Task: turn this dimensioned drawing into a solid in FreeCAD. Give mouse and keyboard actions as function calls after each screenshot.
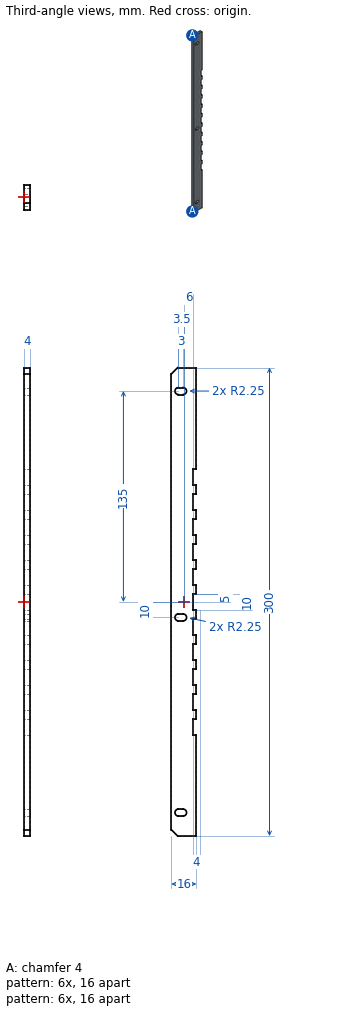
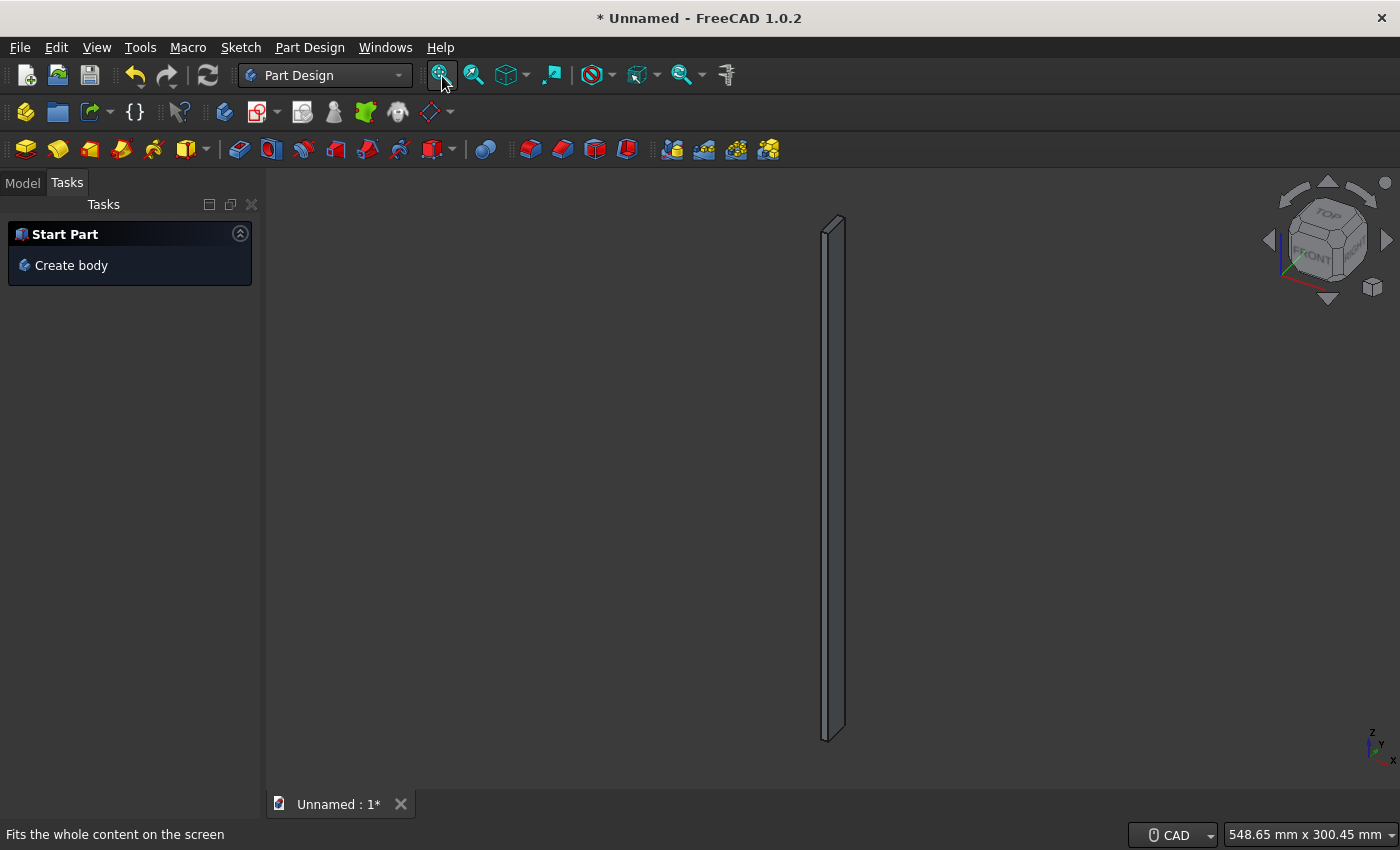
key(0)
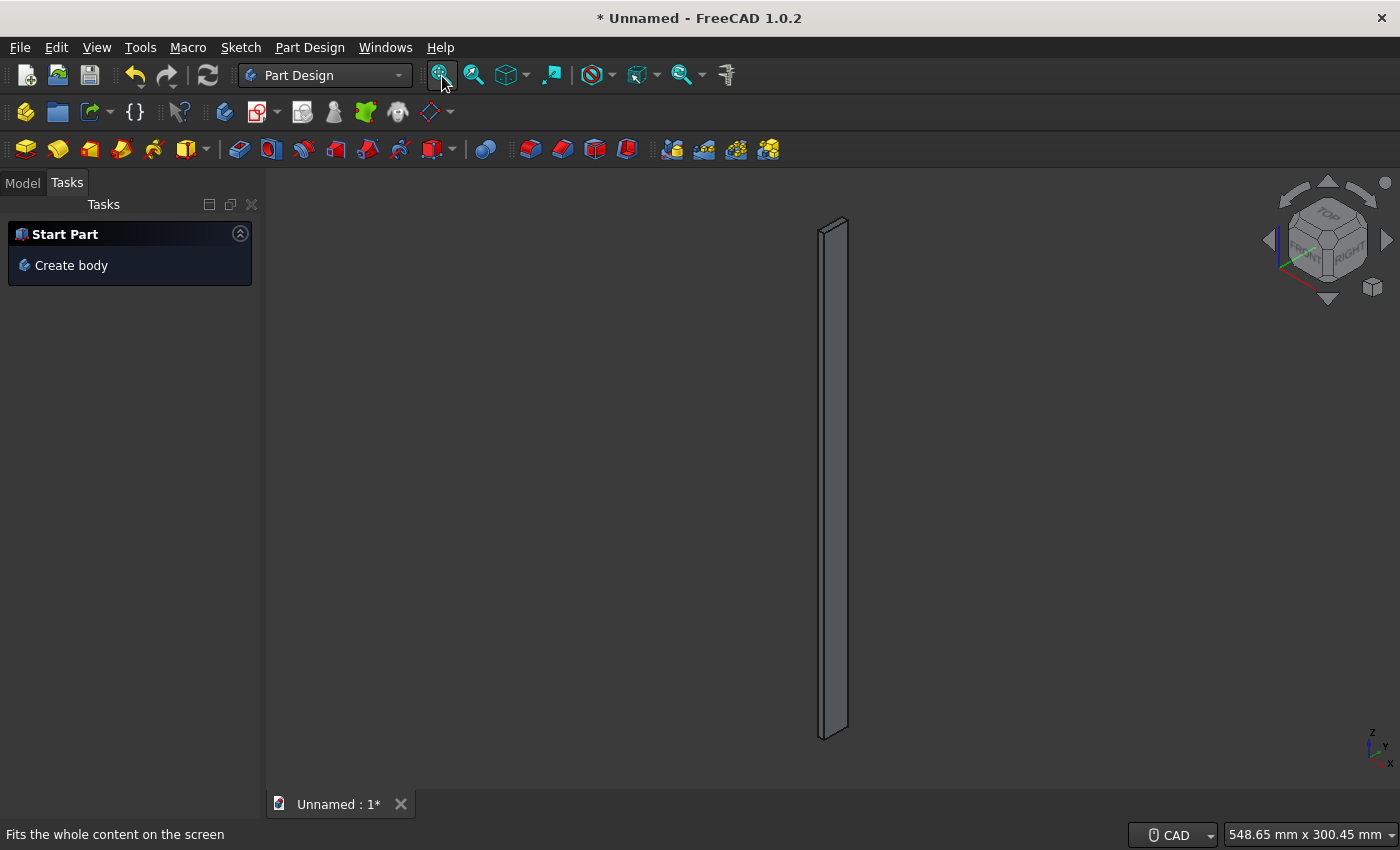
scroll(821, 737, up, 8)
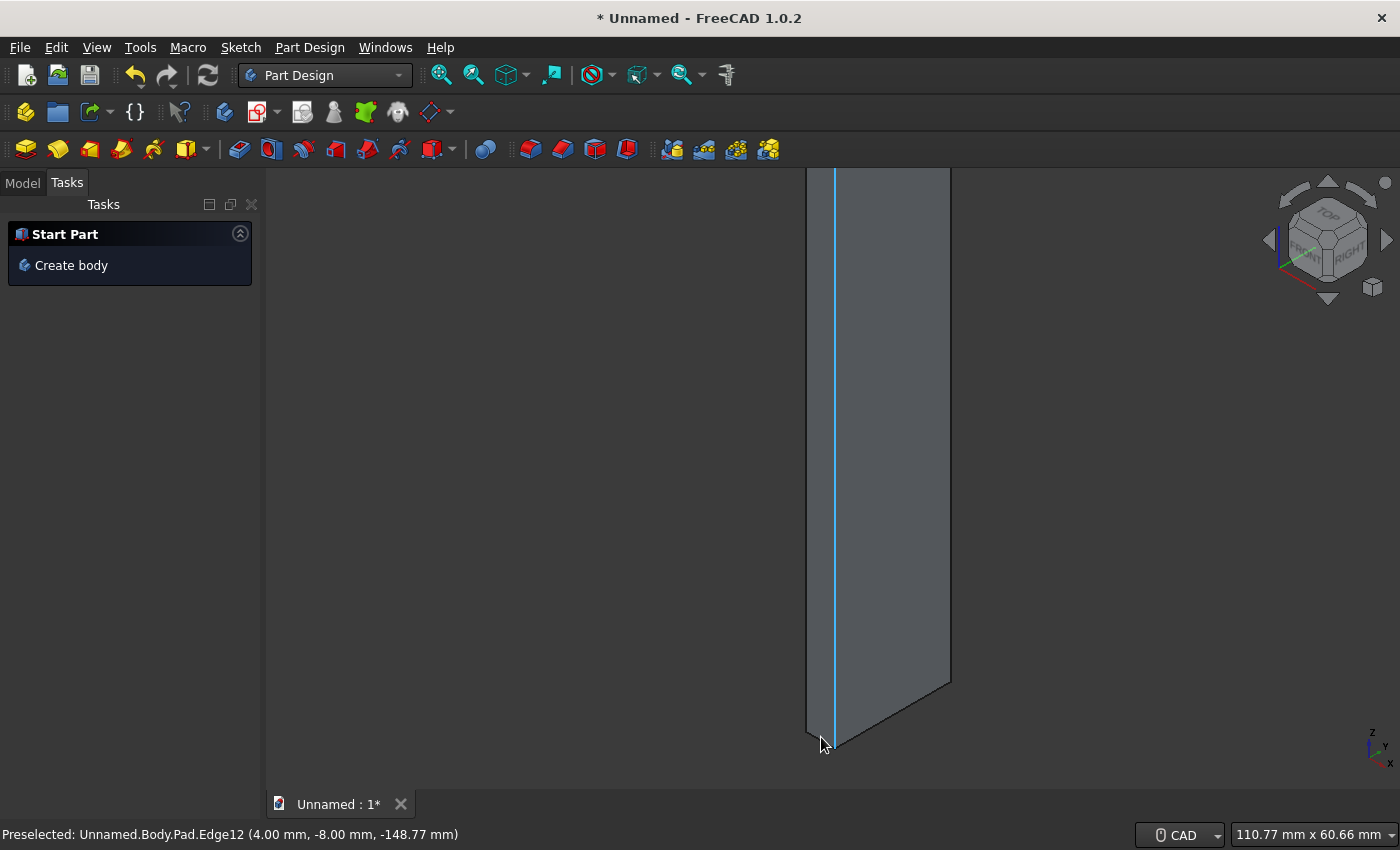
click(442, 76)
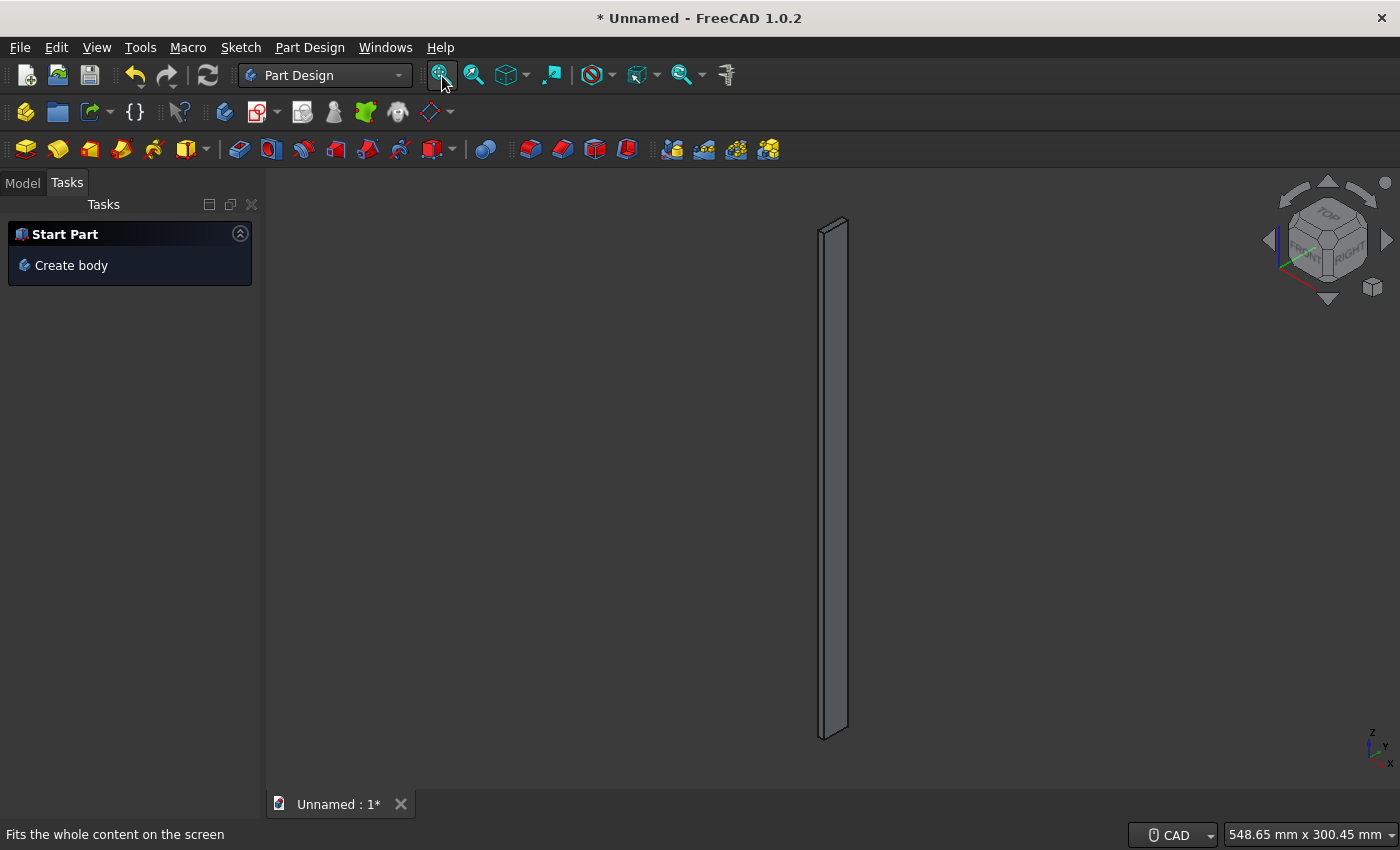
key(2)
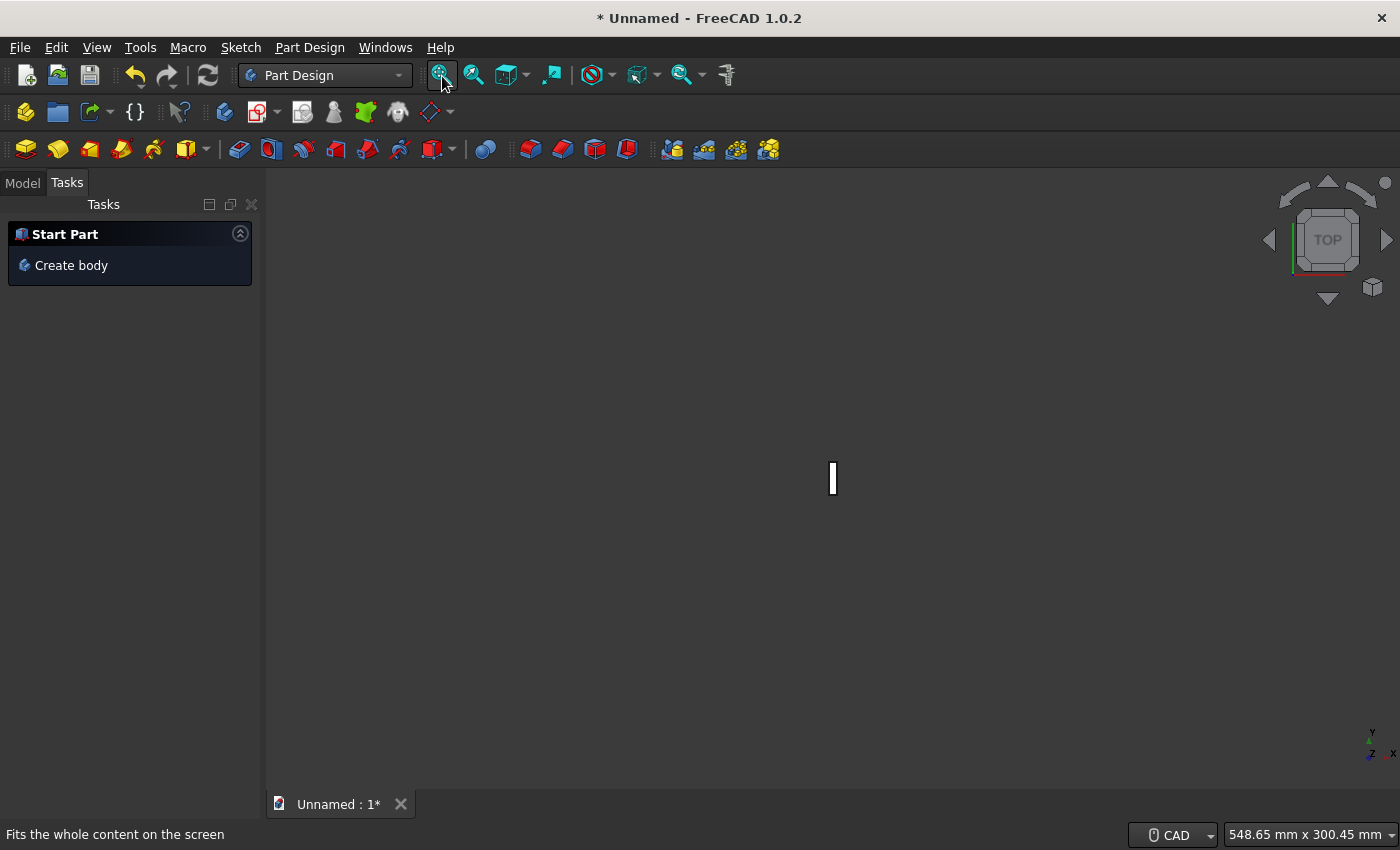
key(v)
key(f)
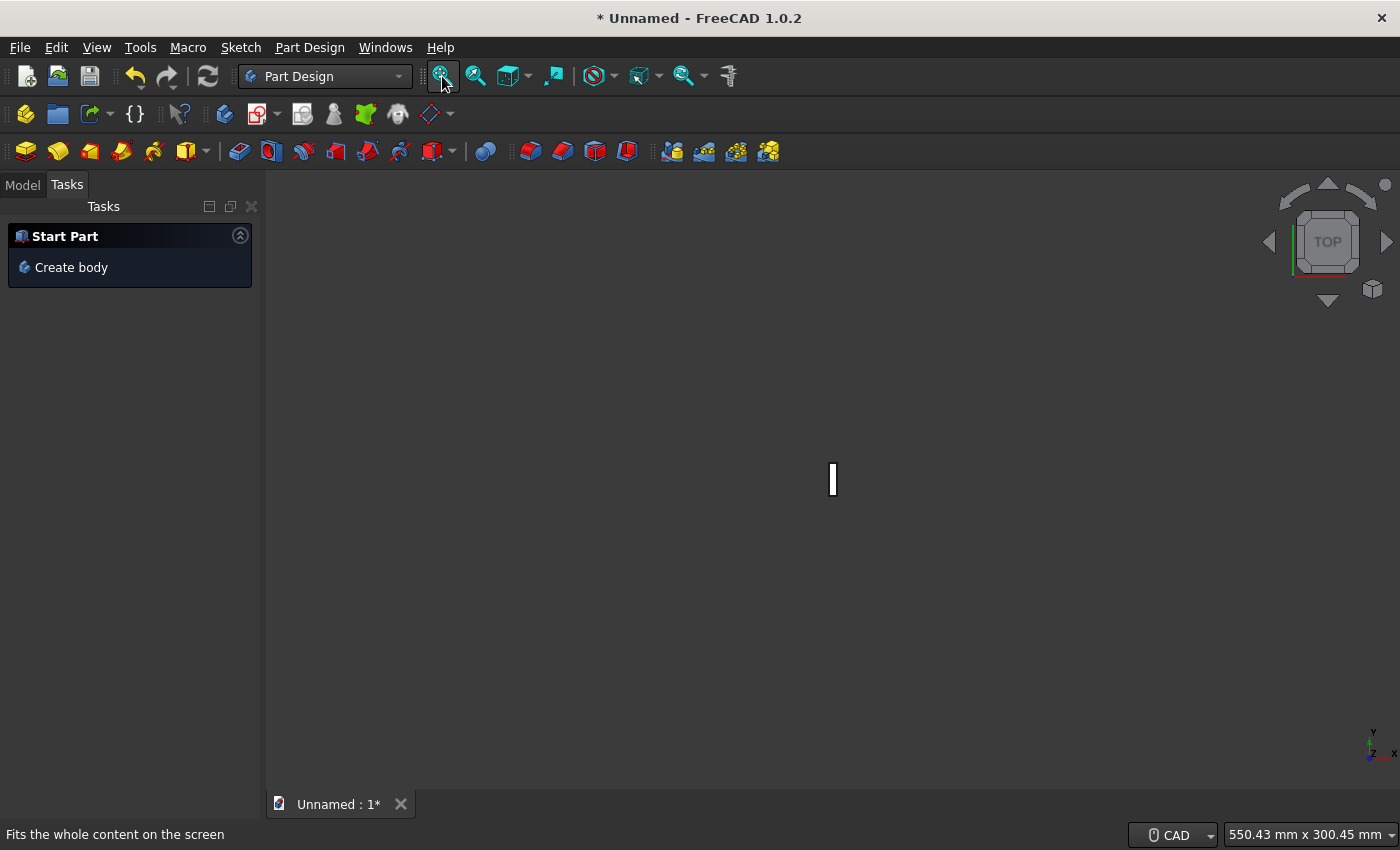
scroll(833, 495, up, 8)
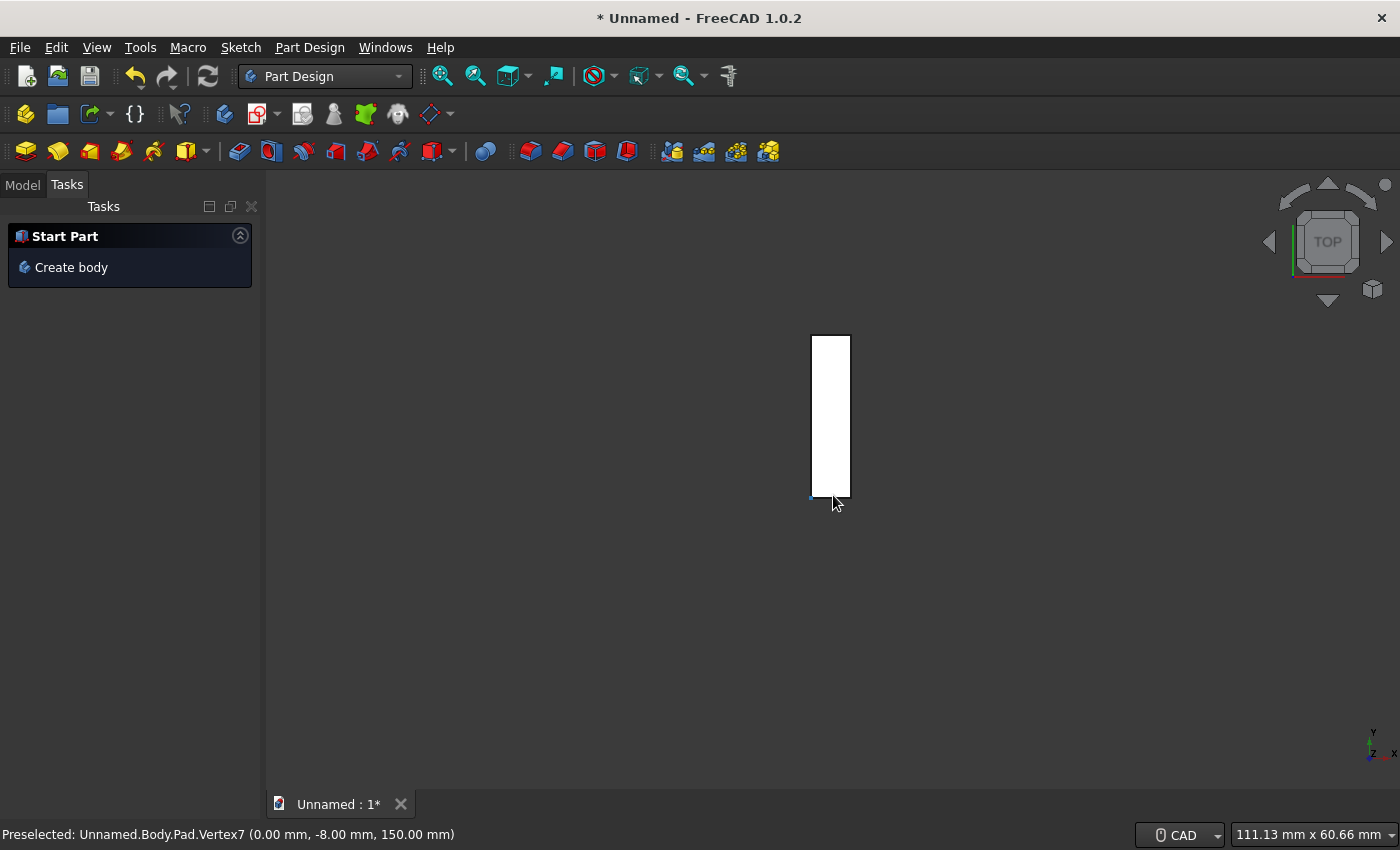
click(831, 497)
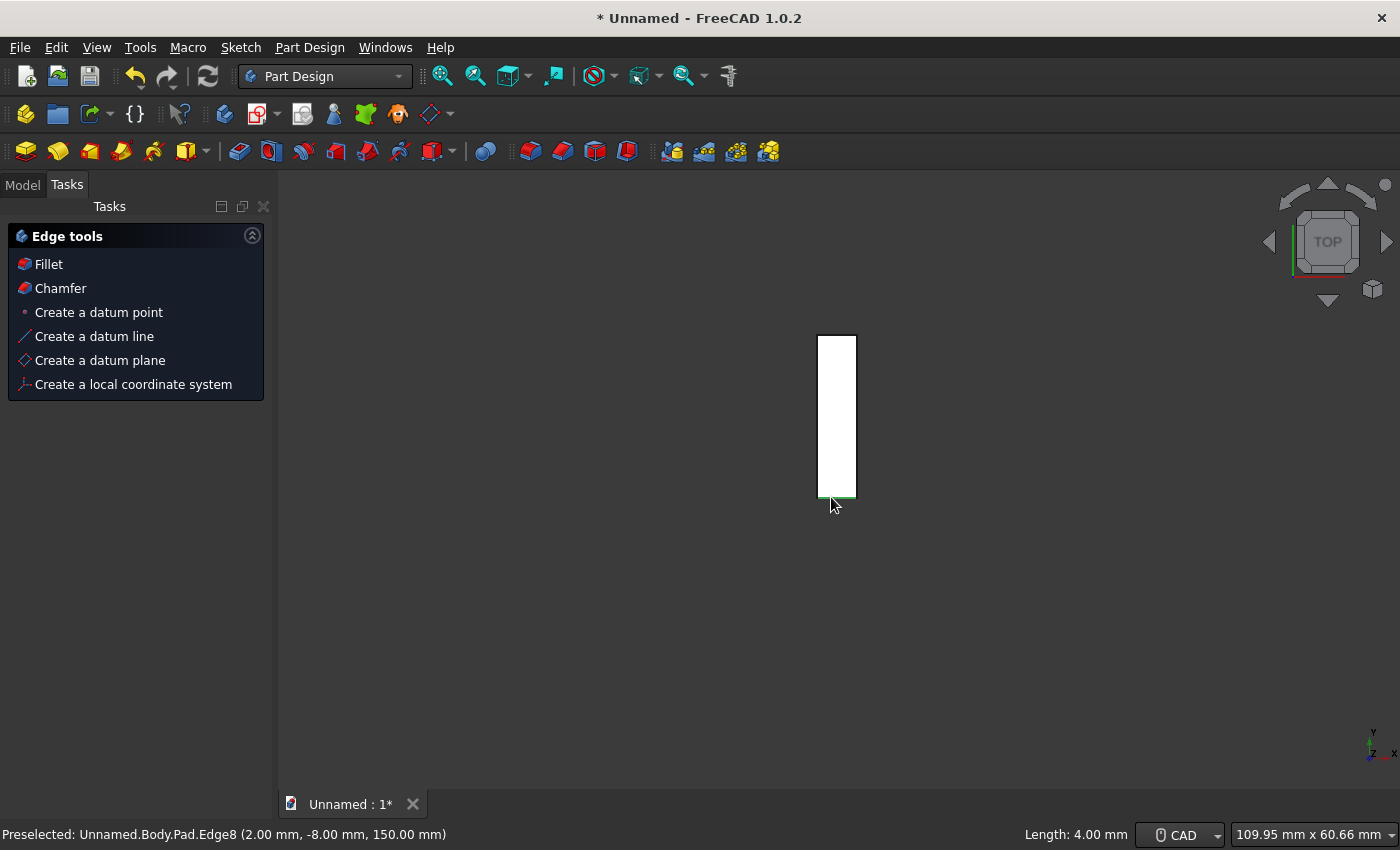
key(v)
key(f)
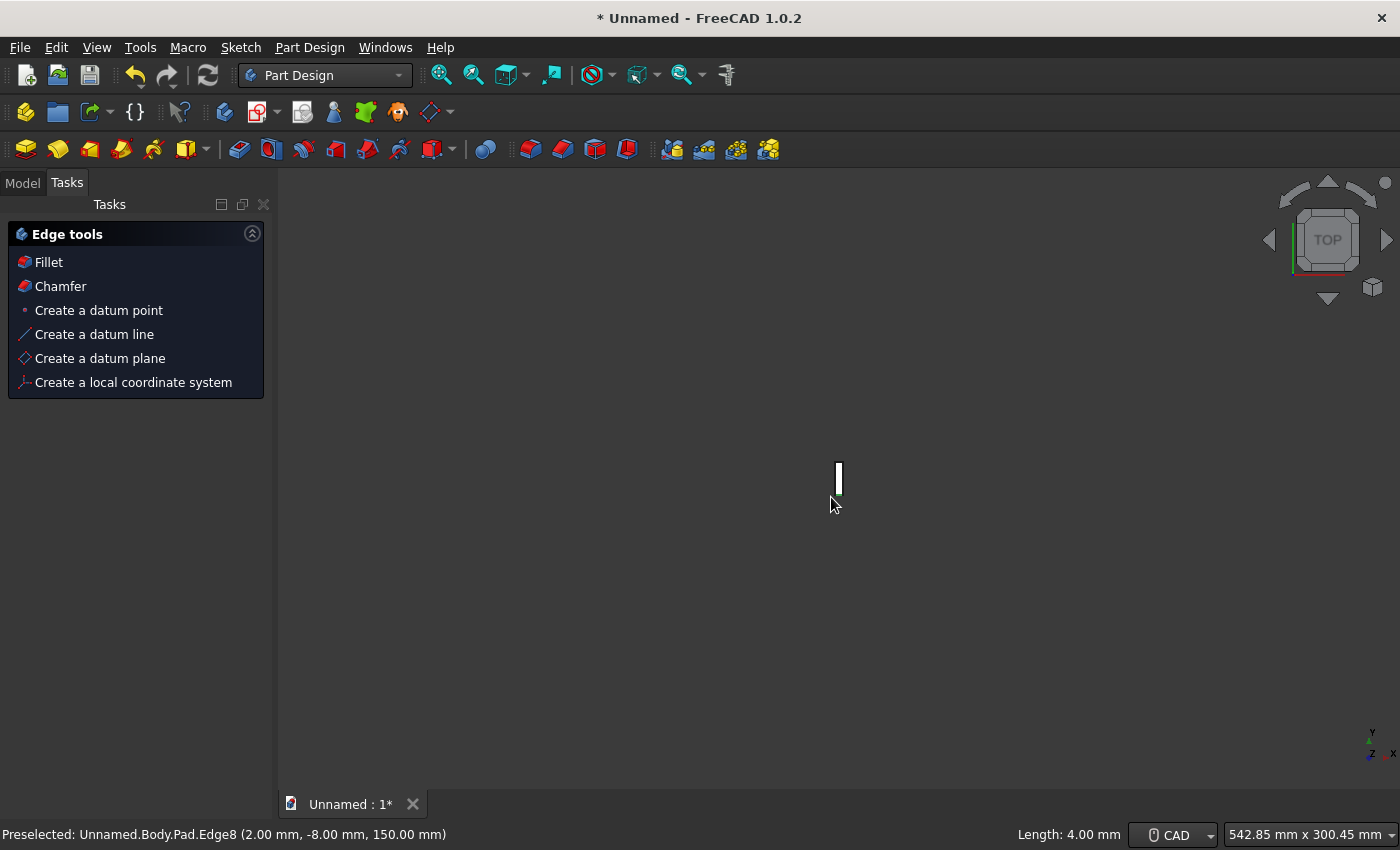
key(1)